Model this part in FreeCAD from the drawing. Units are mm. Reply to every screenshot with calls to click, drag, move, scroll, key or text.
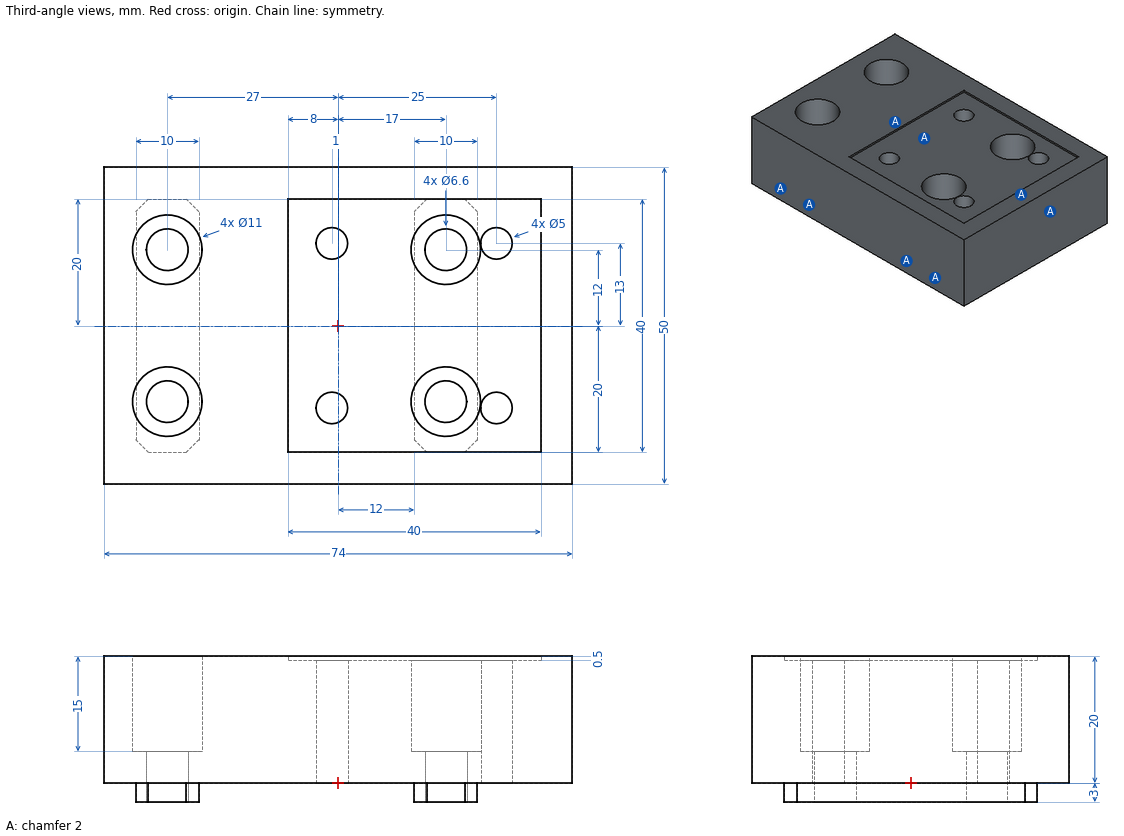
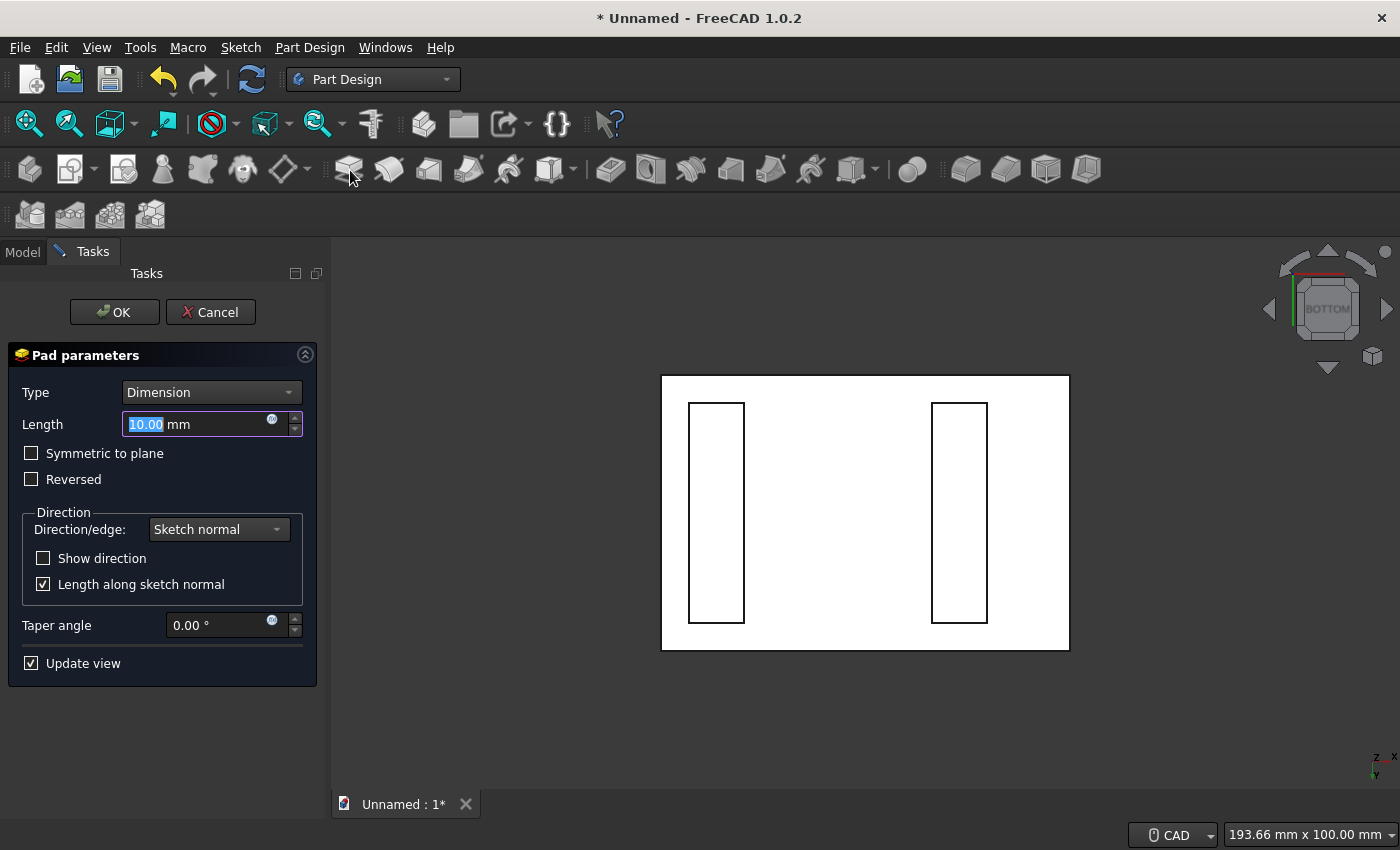
text(3)
key(Tab)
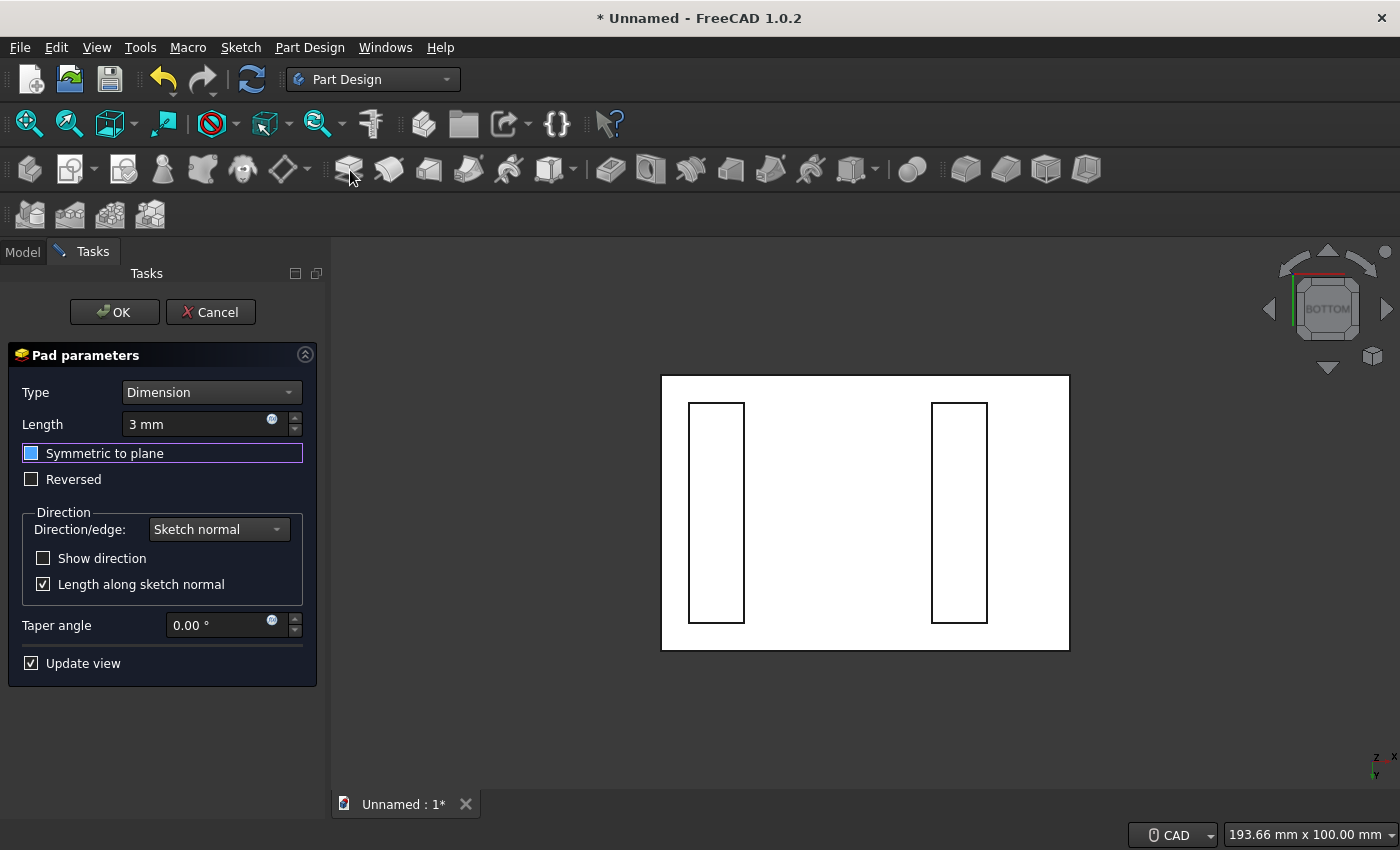
click(115, 312)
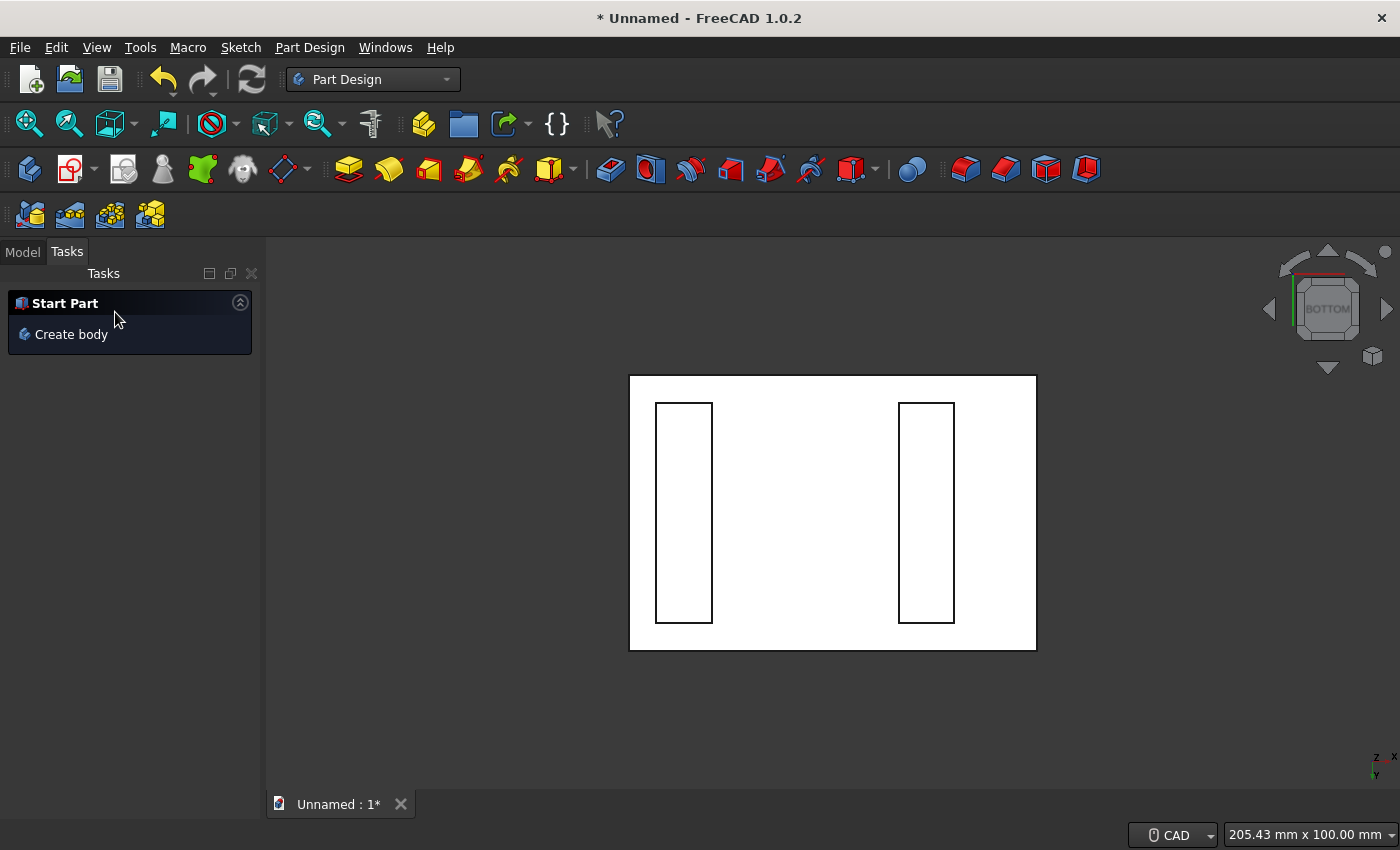
scroll(954, 622, up, 5)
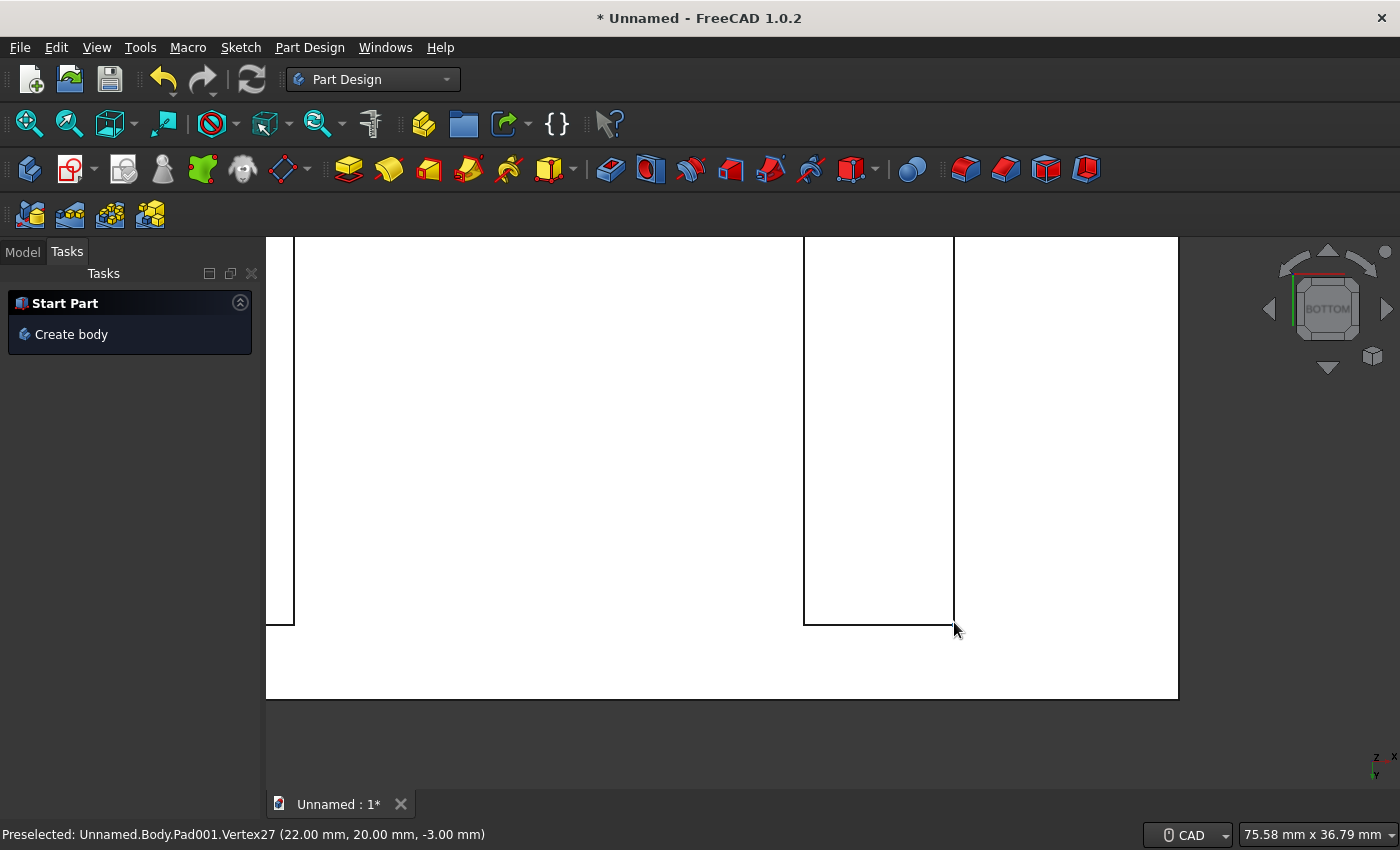
click(30, 124)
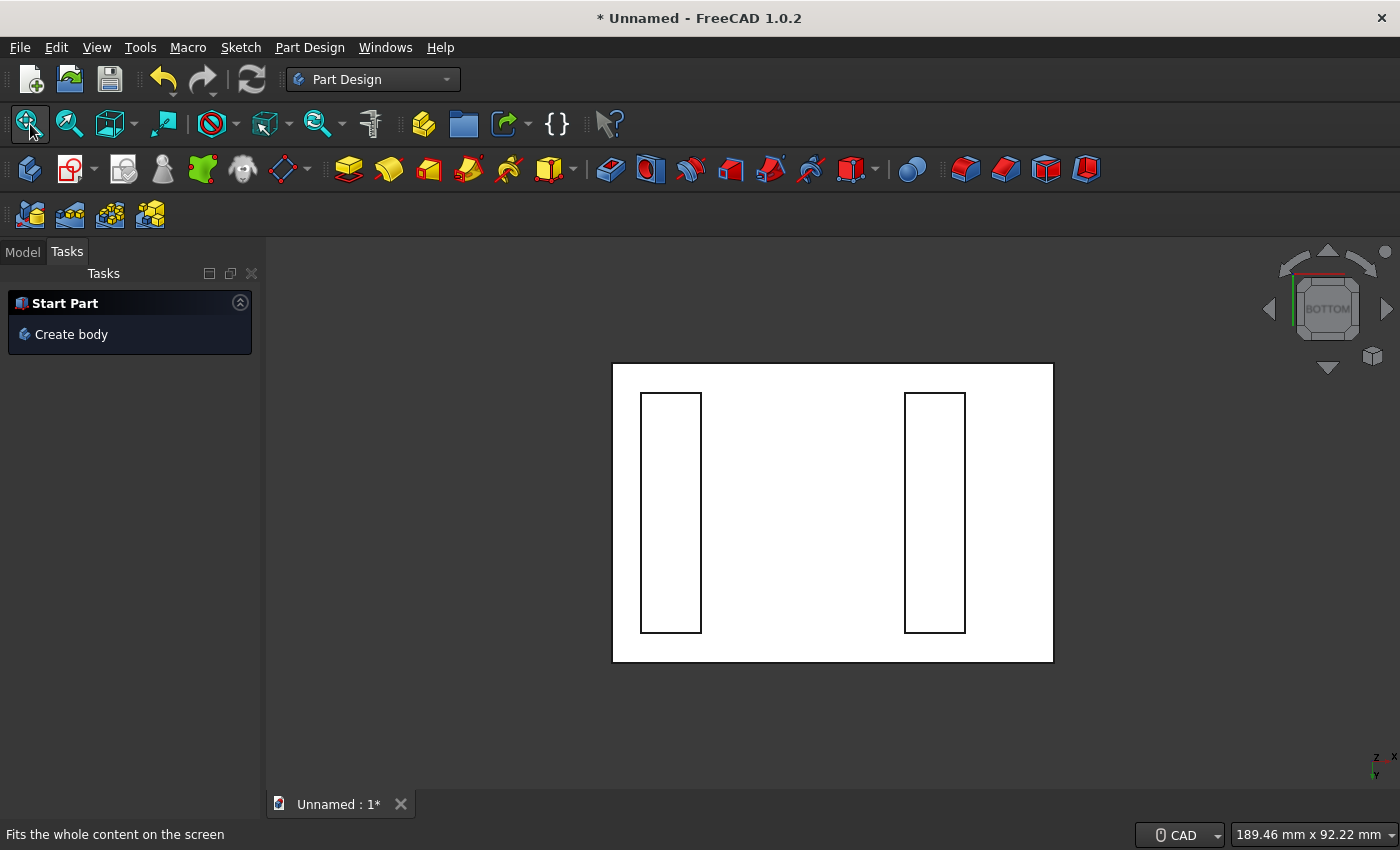
key(0)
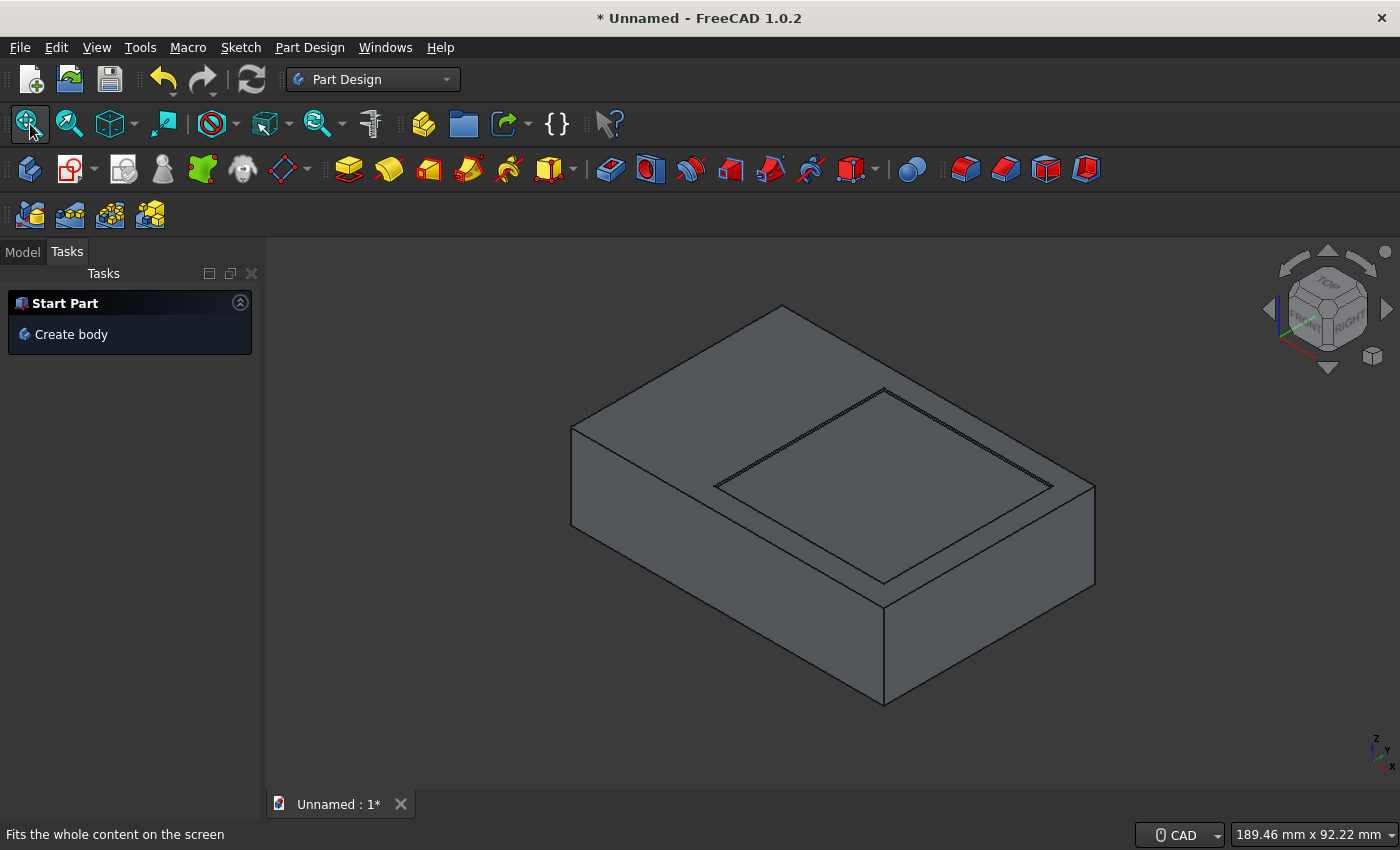
scroll(1011, 566, up, 5)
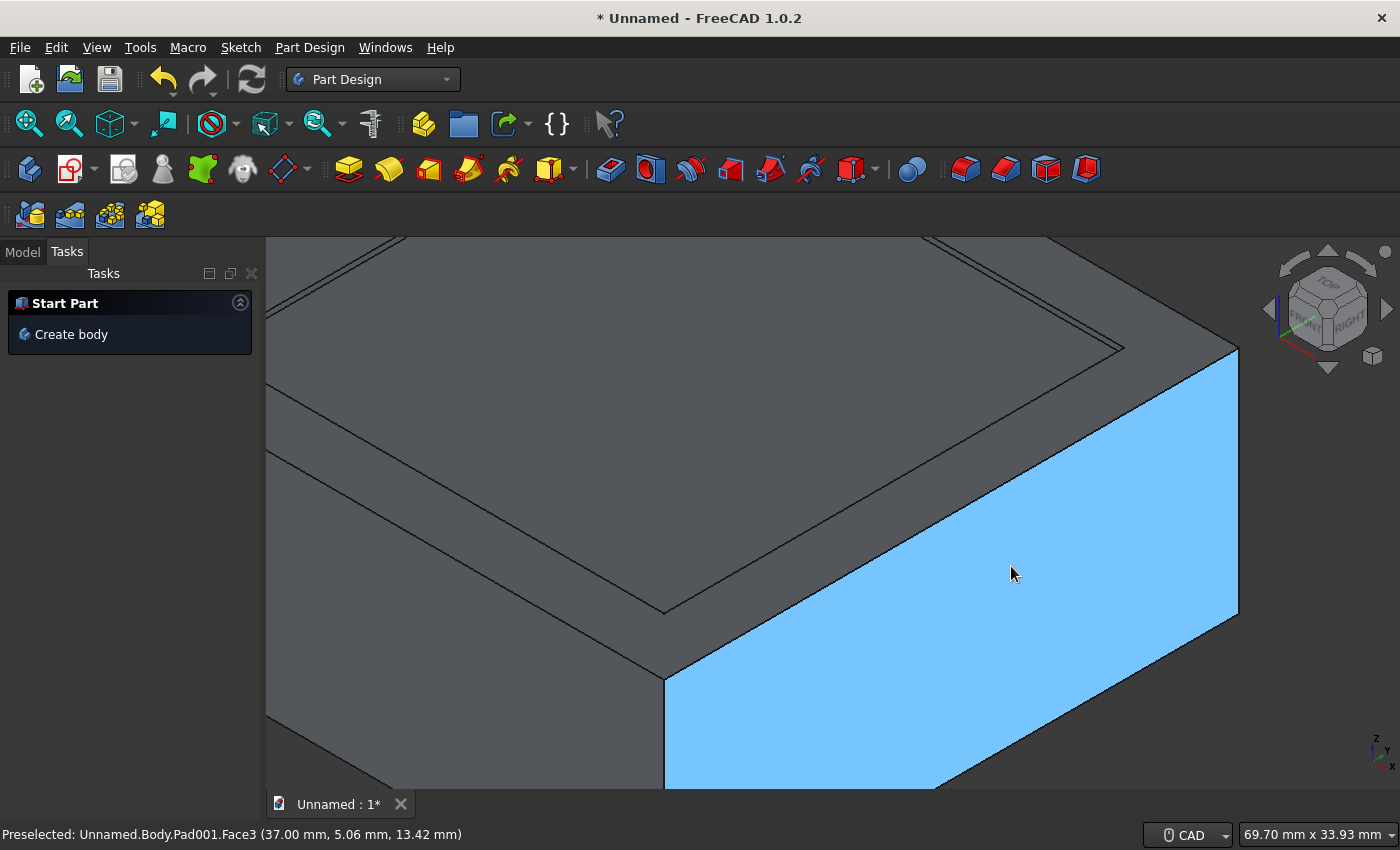
click(30, 124)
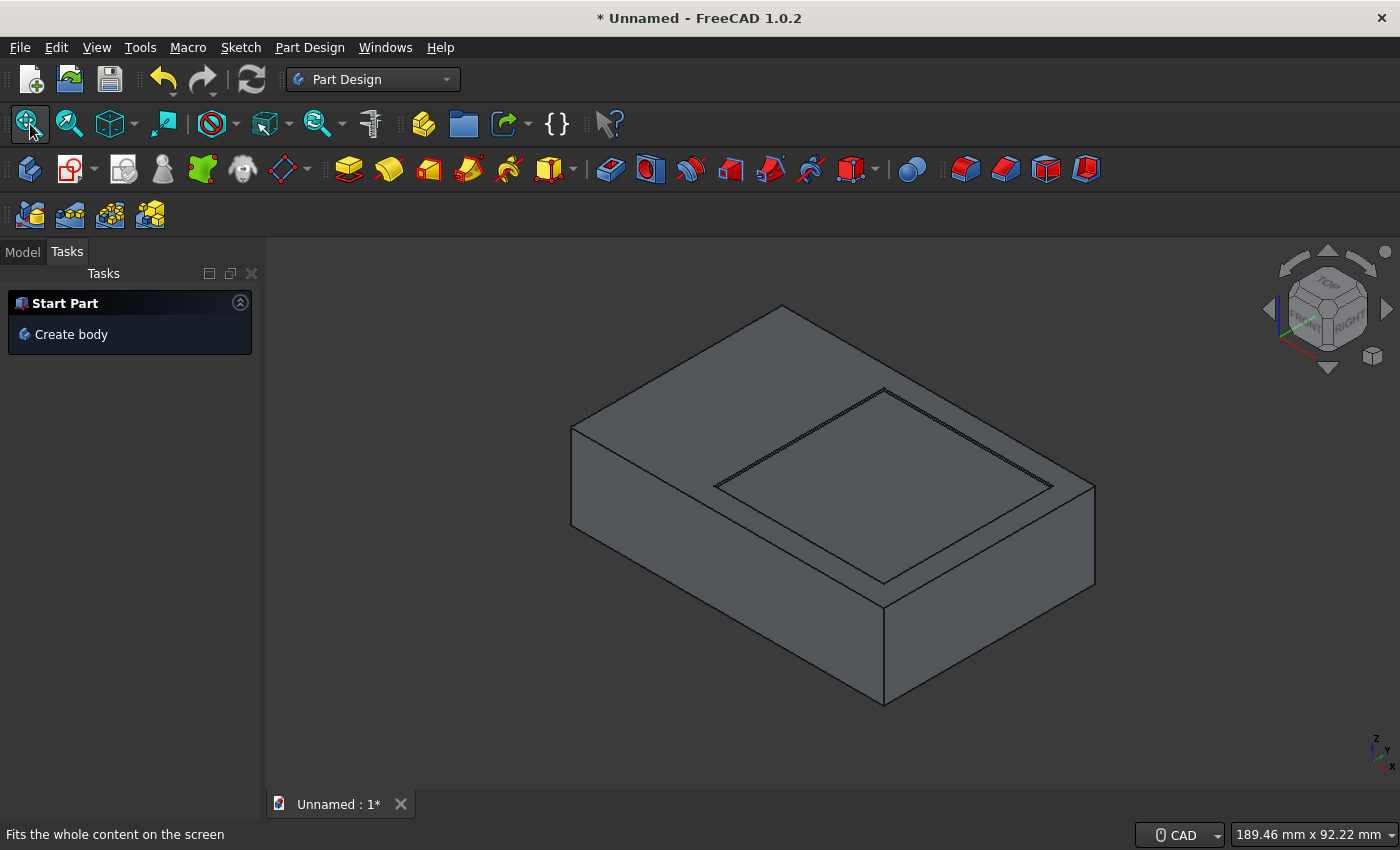
key(2)